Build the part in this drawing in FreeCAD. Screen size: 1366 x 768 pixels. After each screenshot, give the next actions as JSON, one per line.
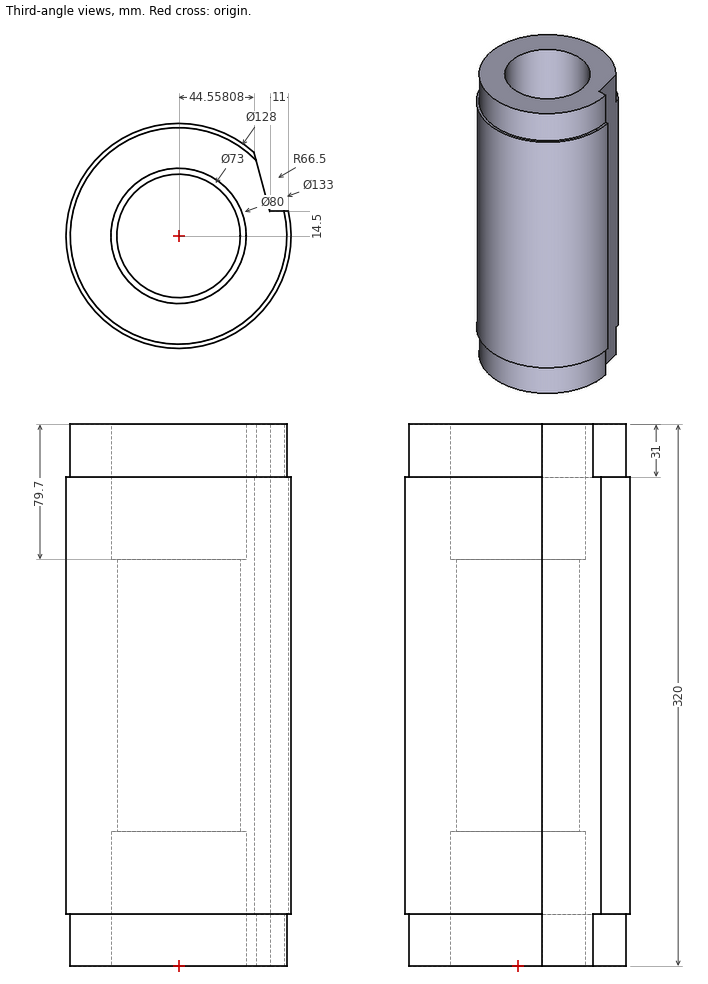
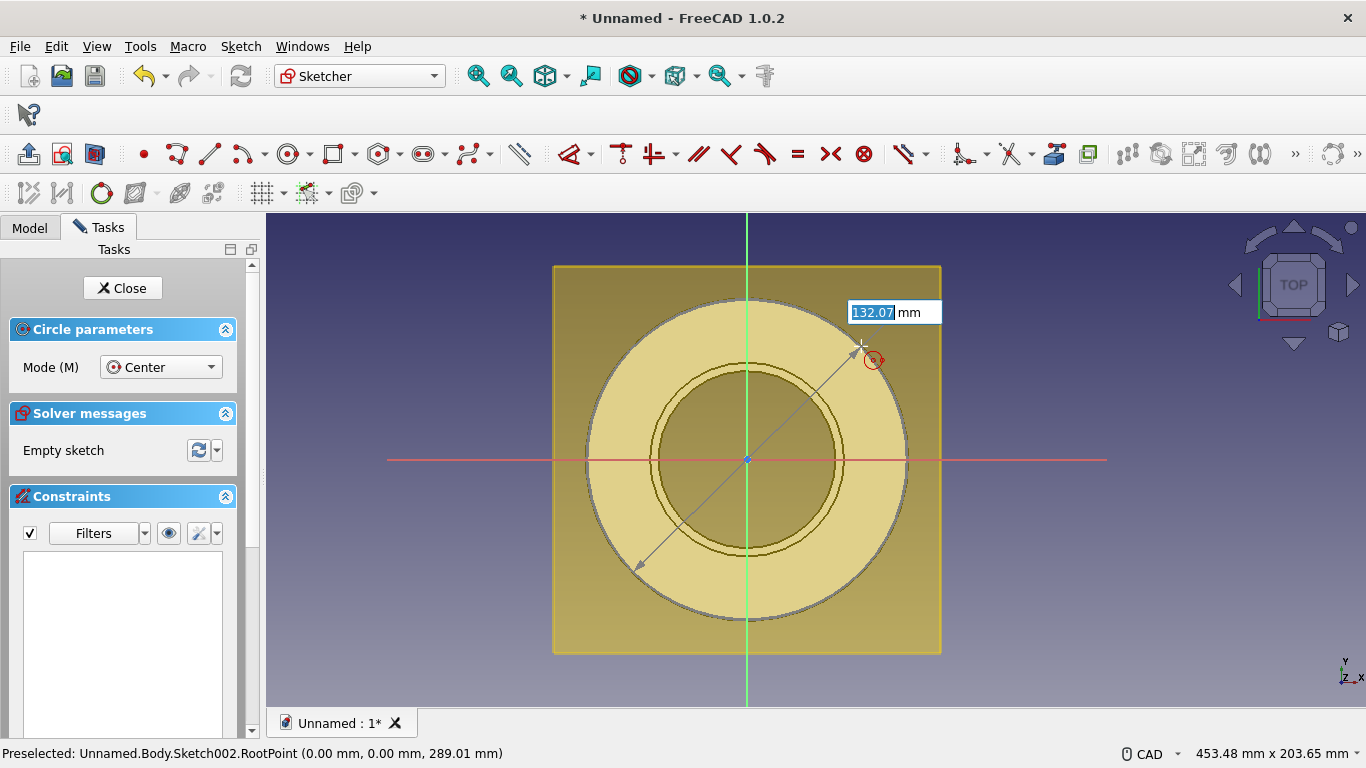
{"action": "type", "text": "133"}
{"action": "key", "text": "Return"}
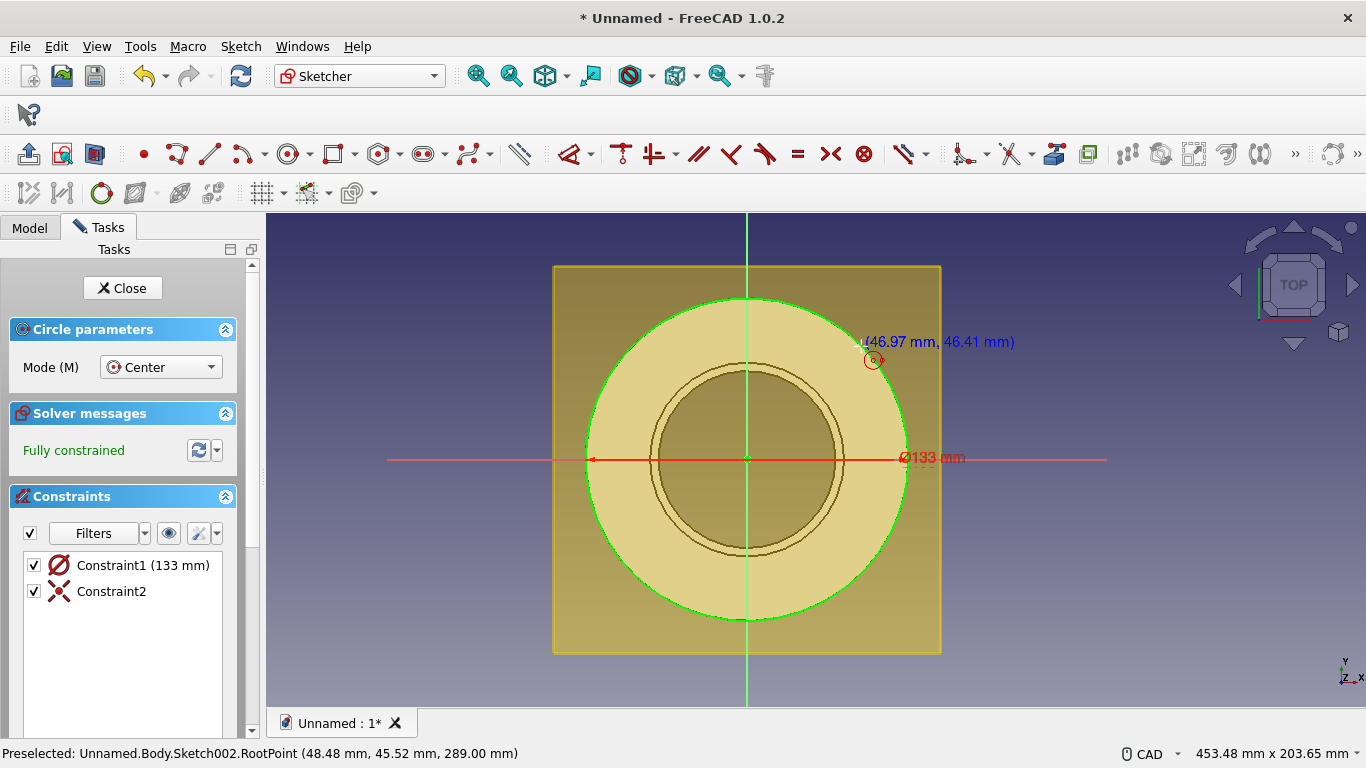
{"action": "left_click", "coordinate": [747, 460]}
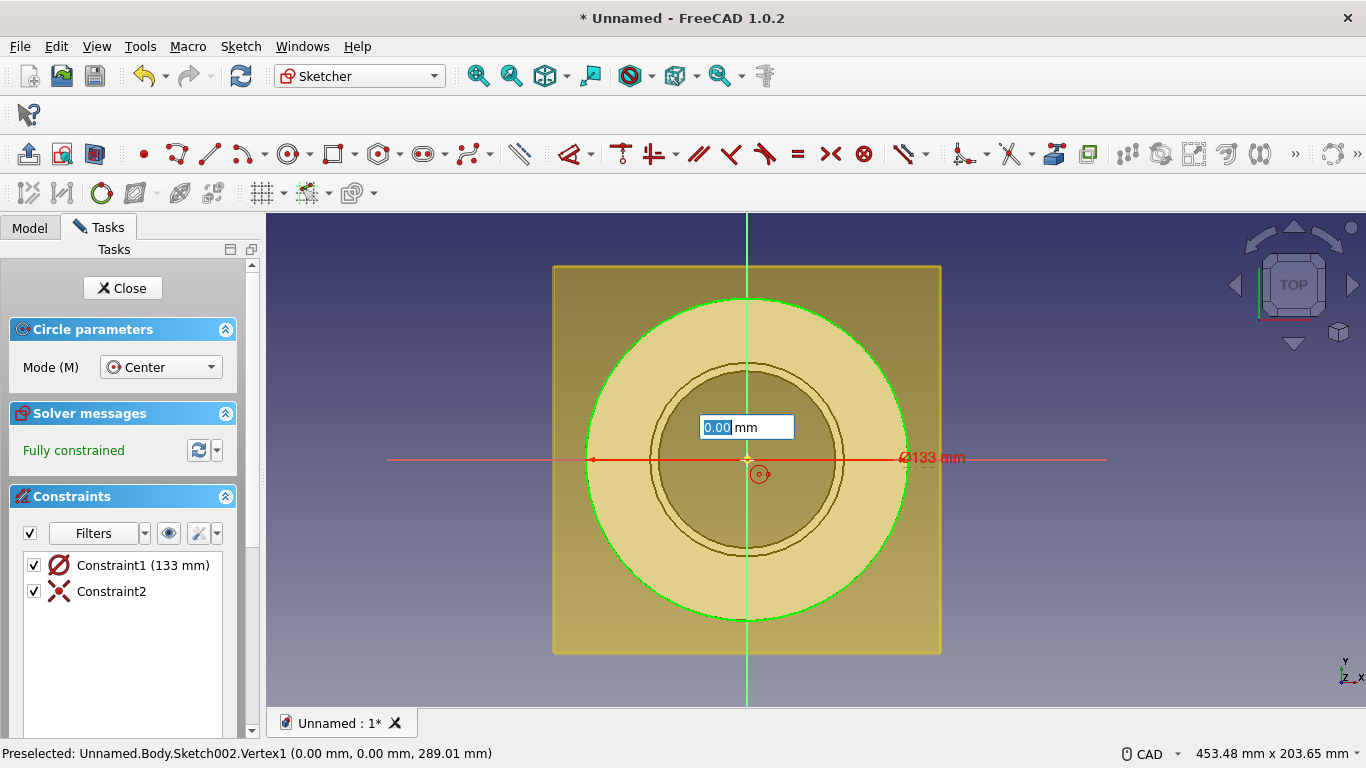
{"action": "scroll", "coordinate": [857, 350], "scroll_direction": "up", "scroll_amount": 5}
{"action": "mouse_move", "coordinate": [856, 349]}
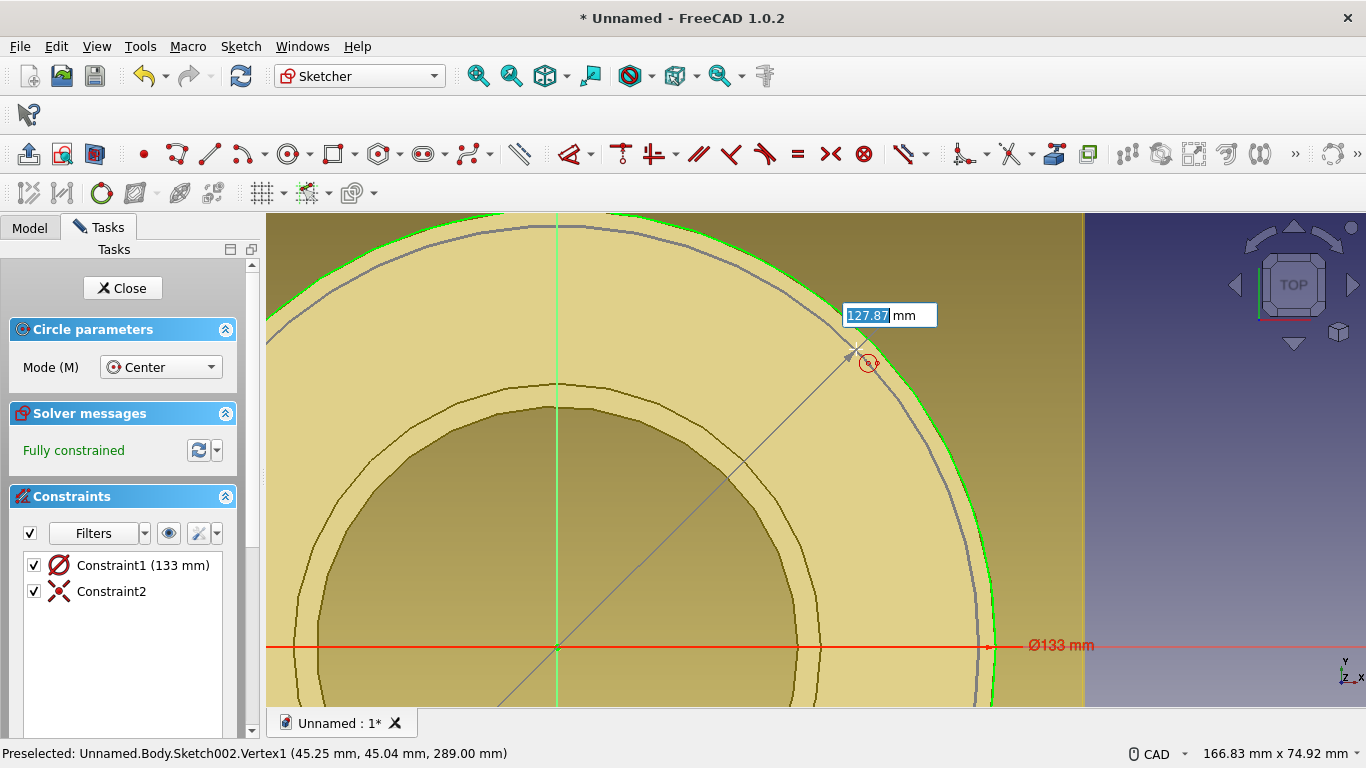
{"action": "type", "text": "128"}
{"action": "key", "text": "Return"}
{"action": "key", "text": "Escape"}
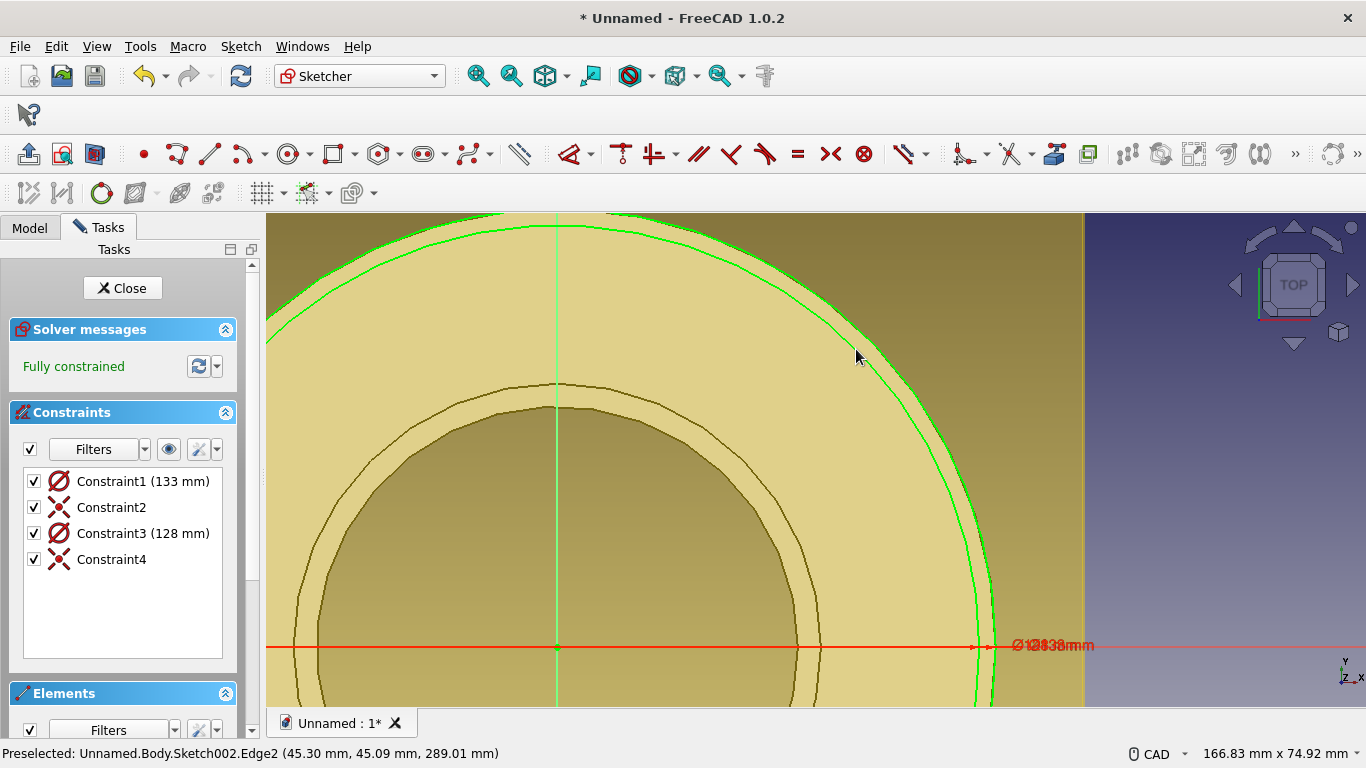
{"action": "left_click", "coordinate": [123, 288]}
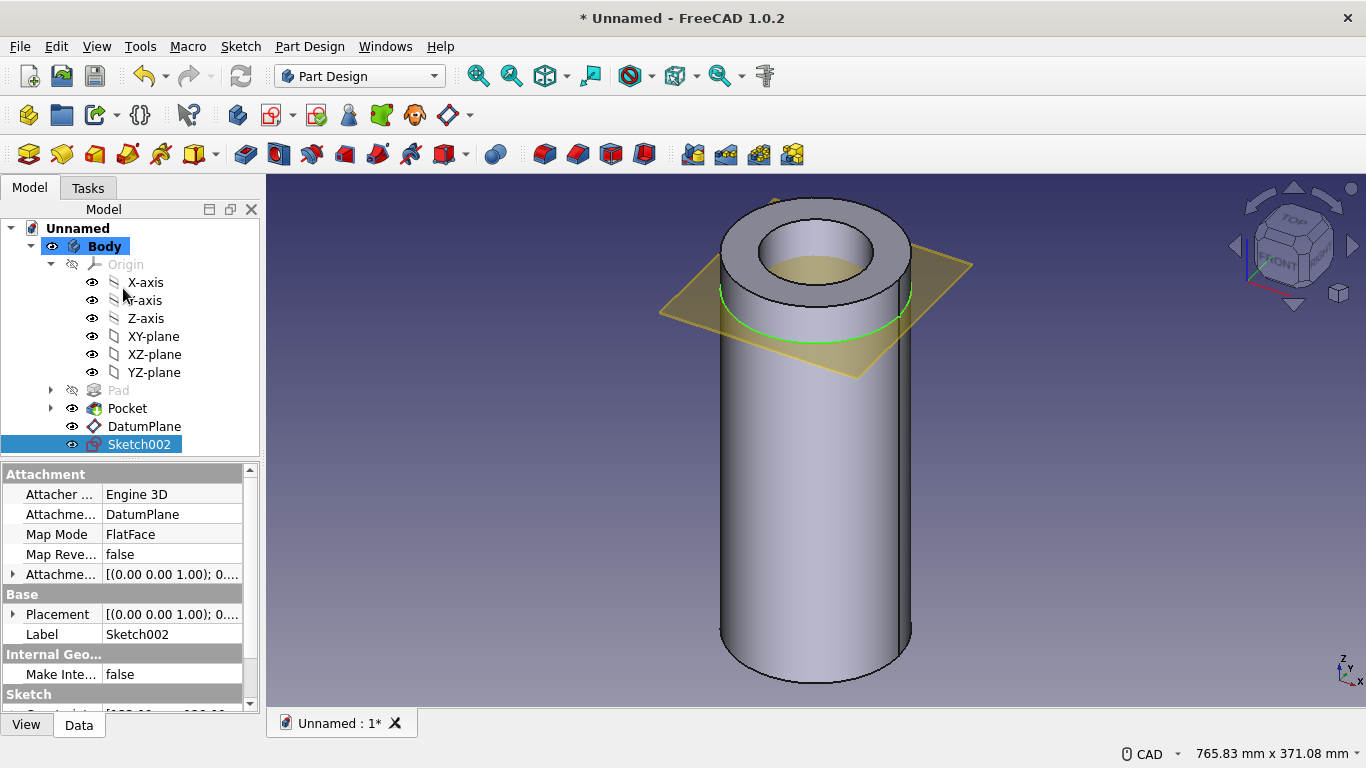
{"action": "left_click", "coordinate": [246, 154]}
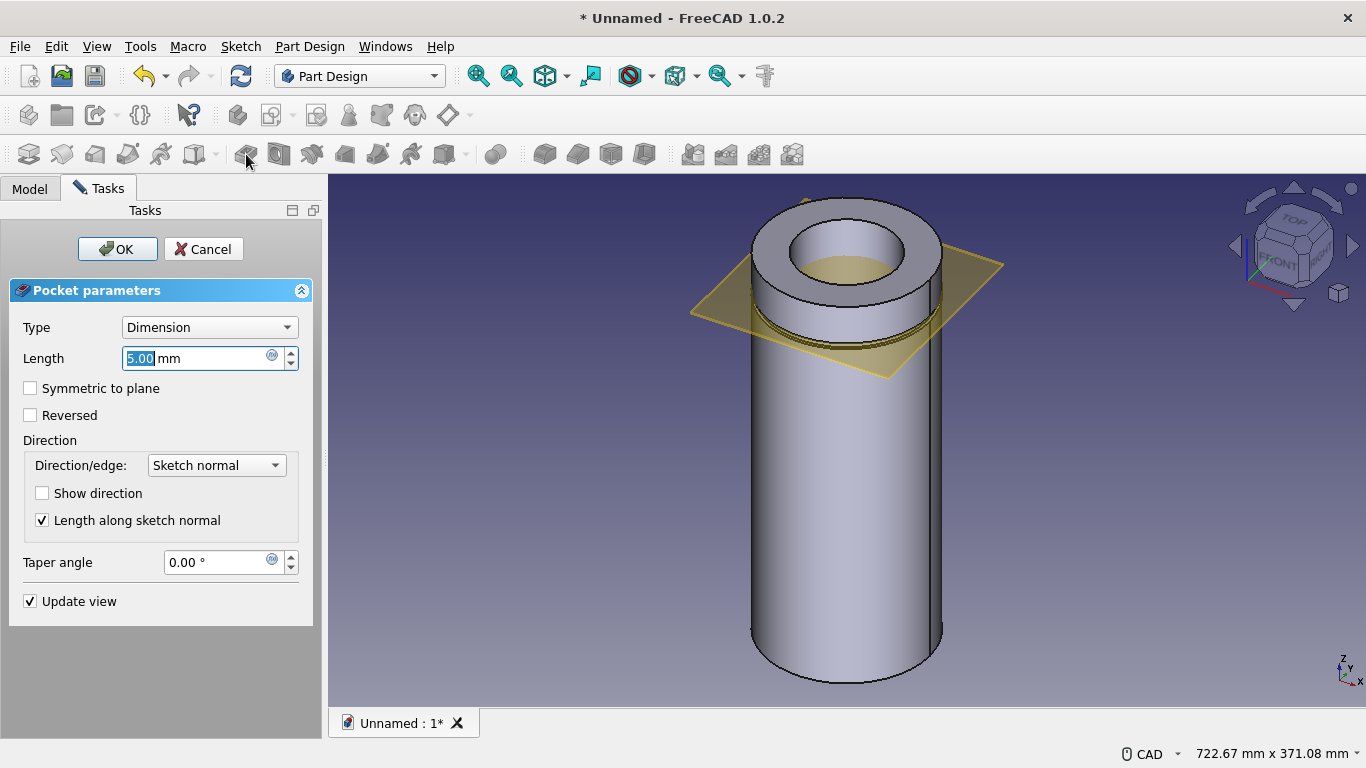
{"action": "type", "text": "31"}
{"action": "key", "text": "Tab"}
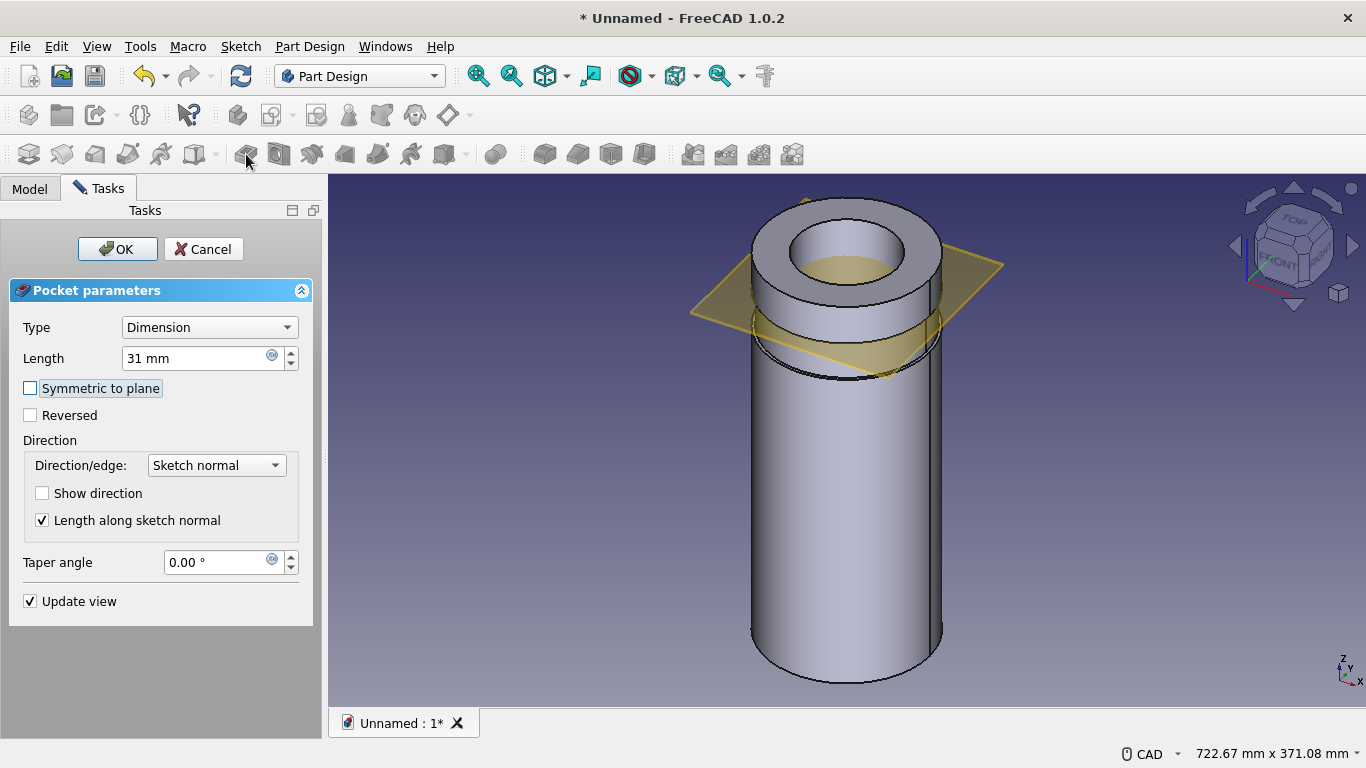
{"action": "left_click", "coordinate": [31, 415]}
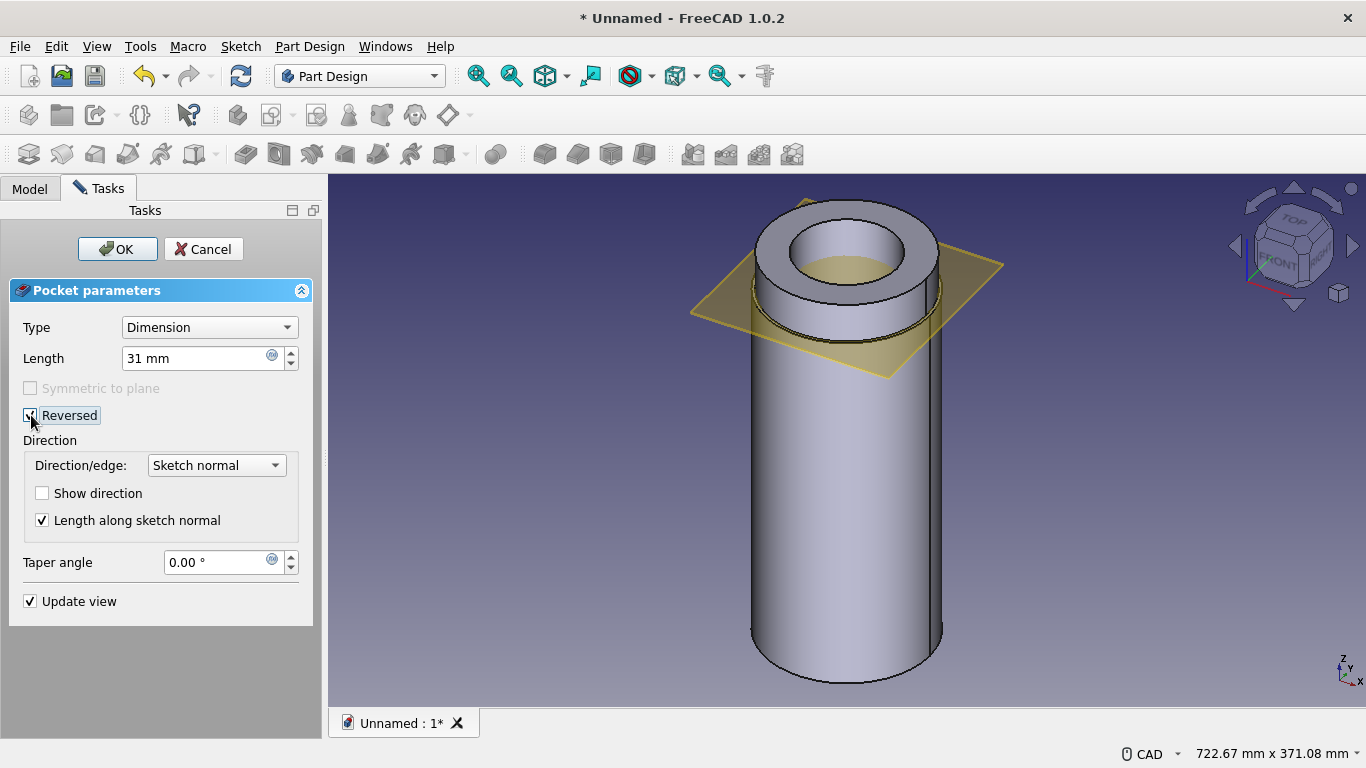
{"action": "left_click", "coordinate": [118, 249]}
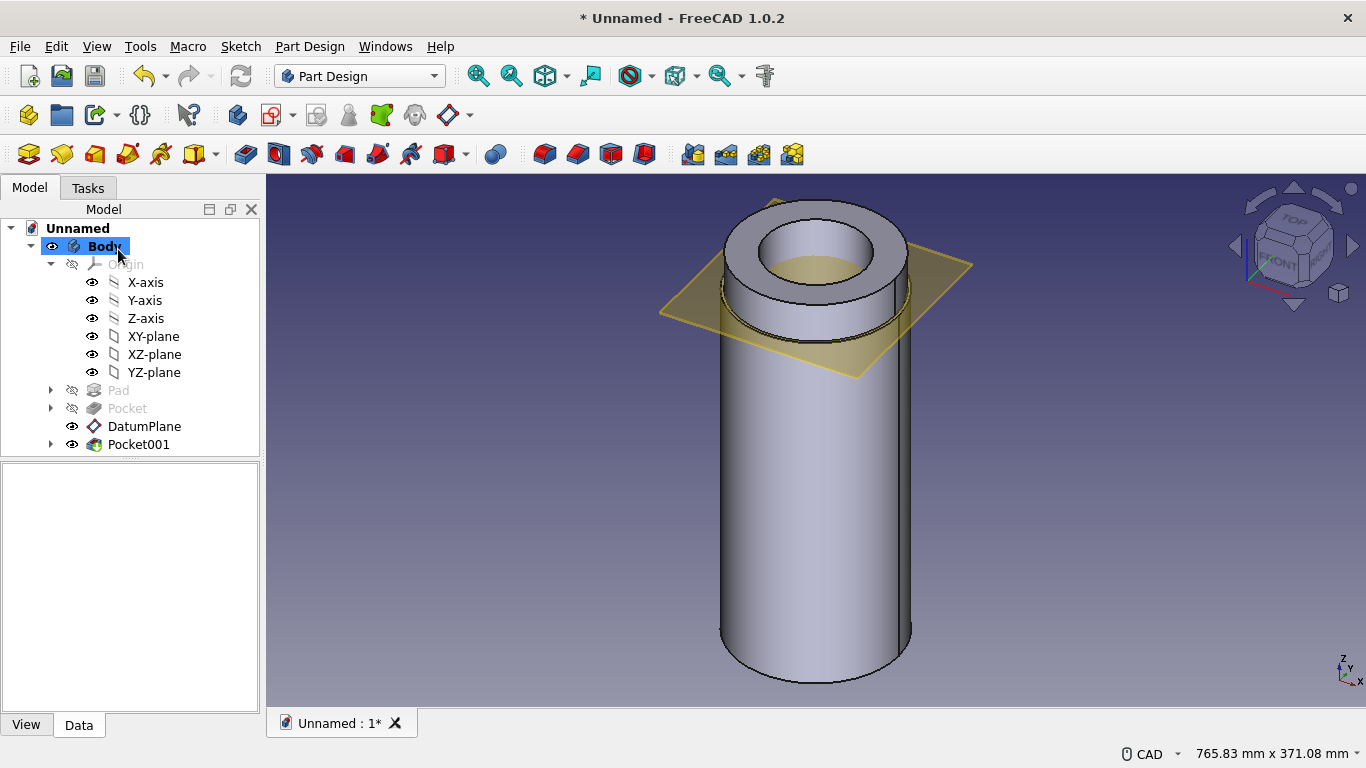
{"action": "left_click", "coordinate": [117, 426]}
{"action": "key", "text": "space"}